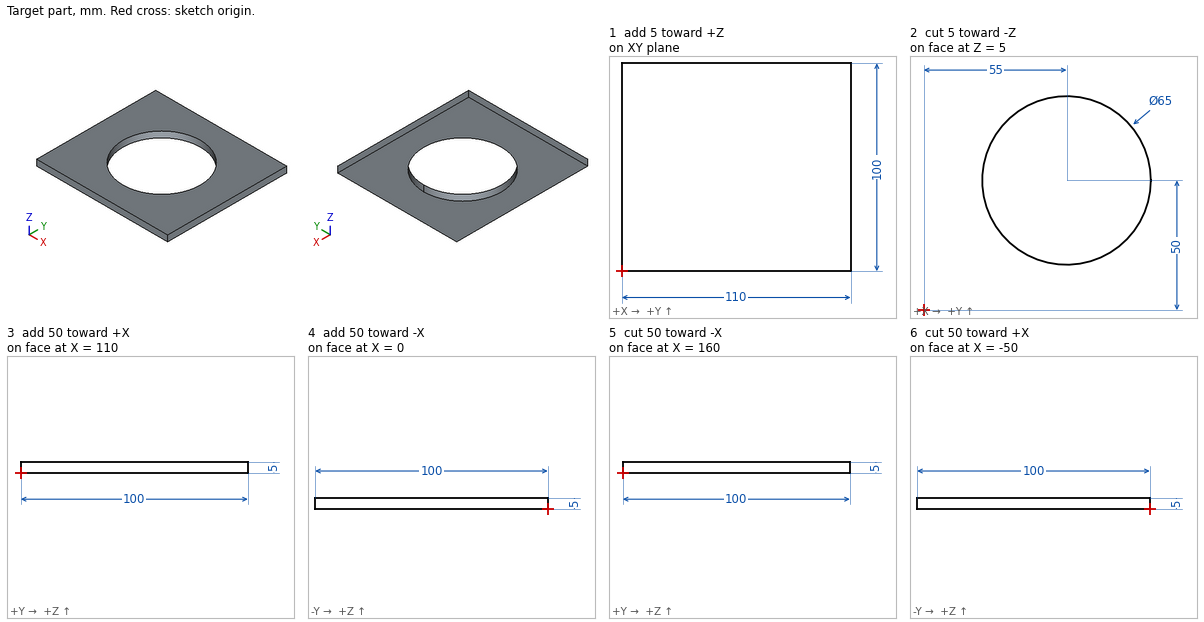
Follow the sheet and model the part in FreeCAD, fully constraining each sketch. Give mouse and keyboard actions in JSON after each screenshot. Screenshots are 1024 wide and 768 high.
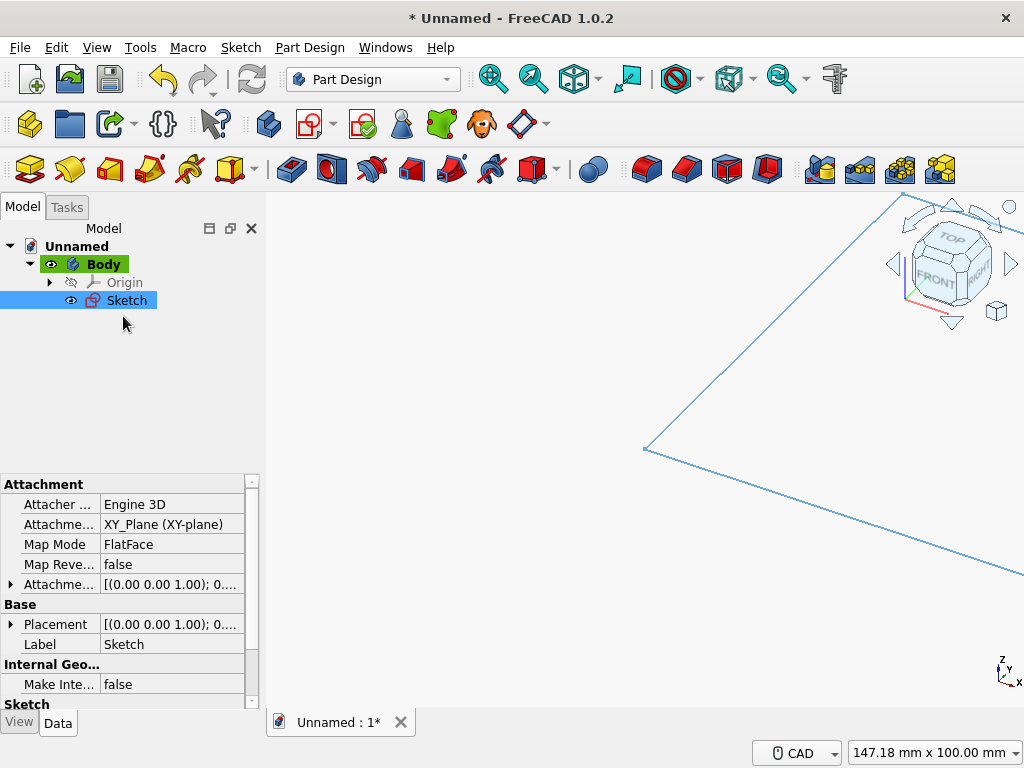
{"action": "left_click", "coordinate": [30, 170]}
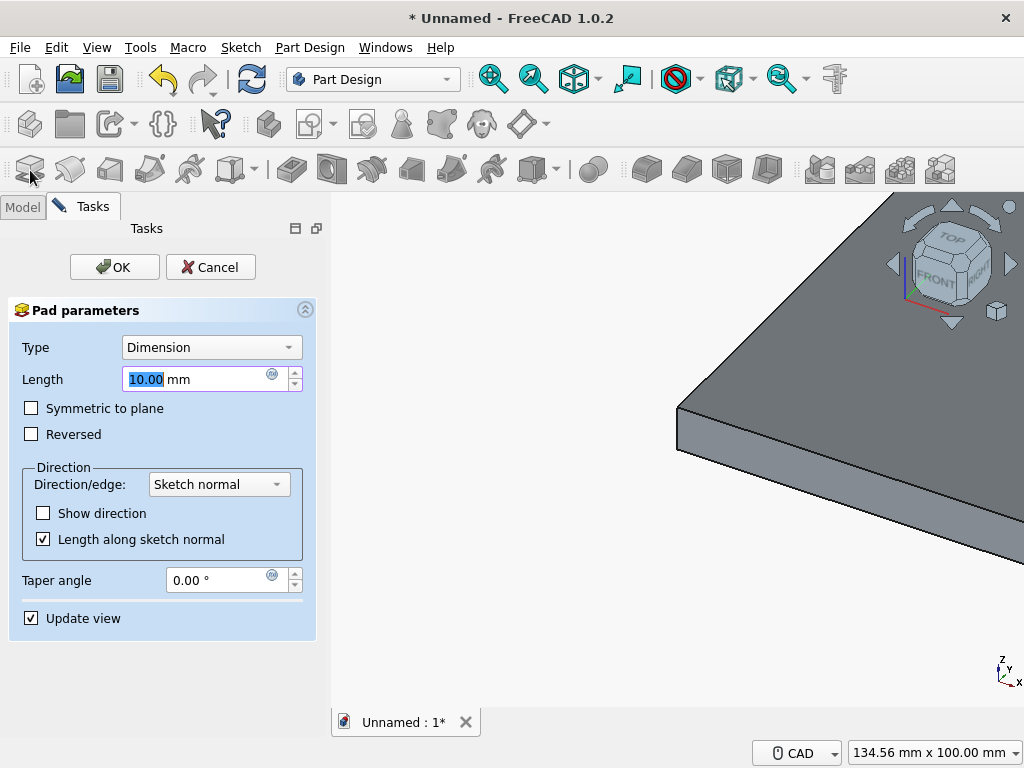
{"action": "type", "text": "5"}
{"action": "key", "text": "Tab"}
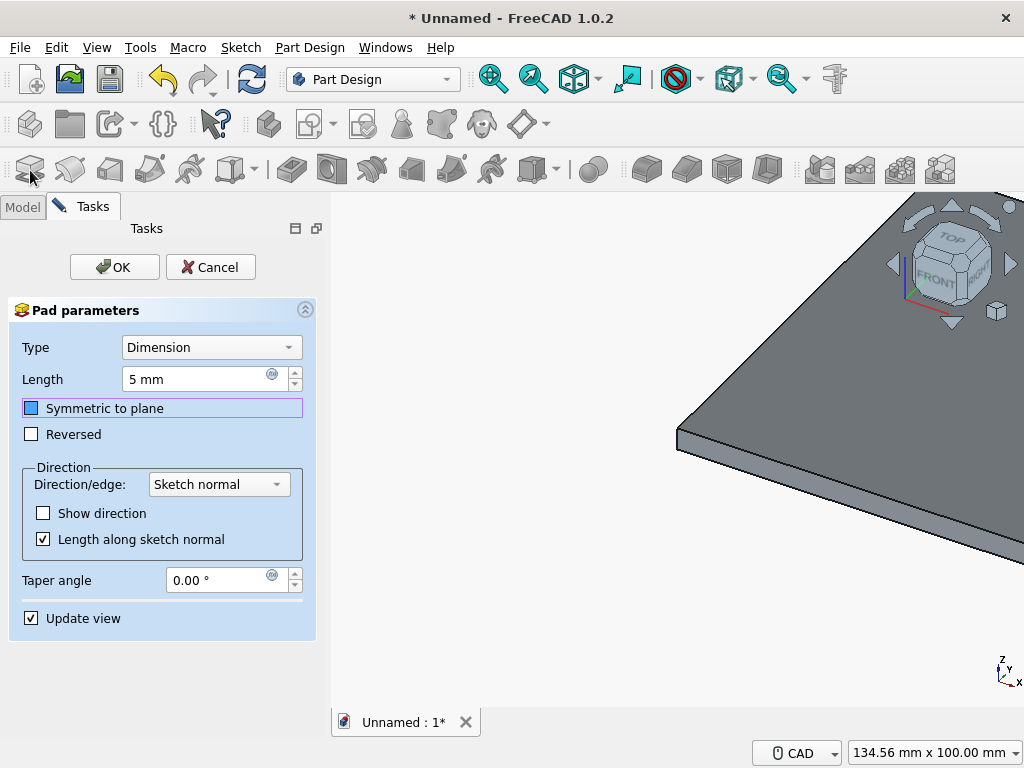
{"action": "left_click", "coordinate": [115, 267]}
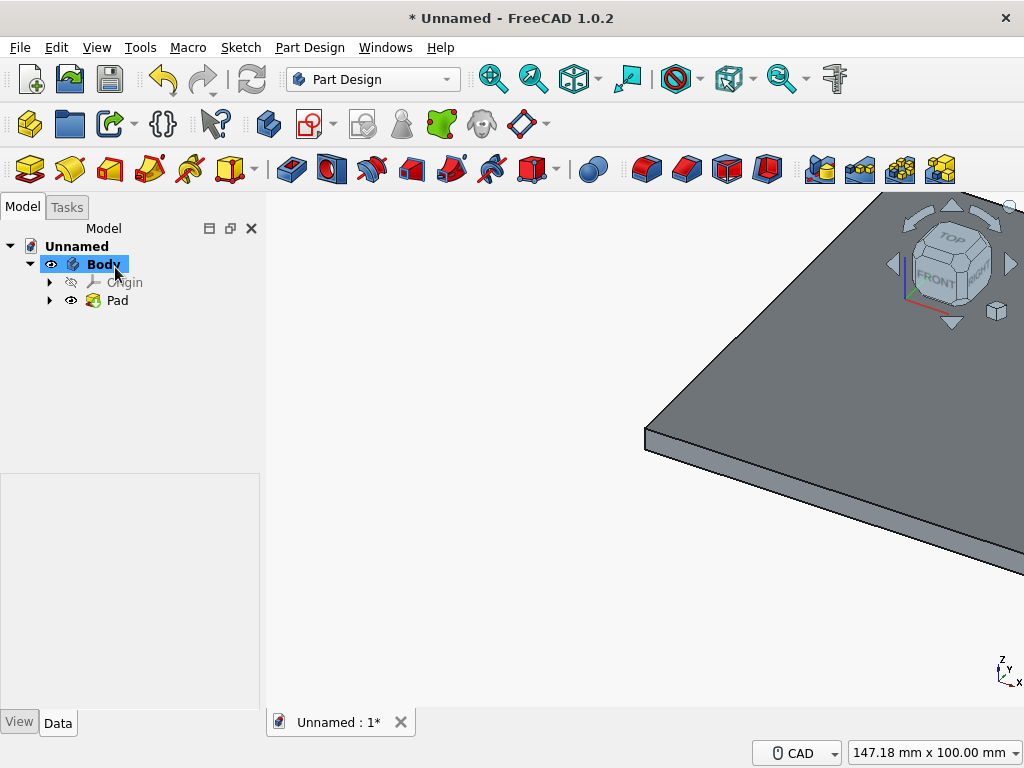
{"action": "left_click", "coordinate": [494, 80]}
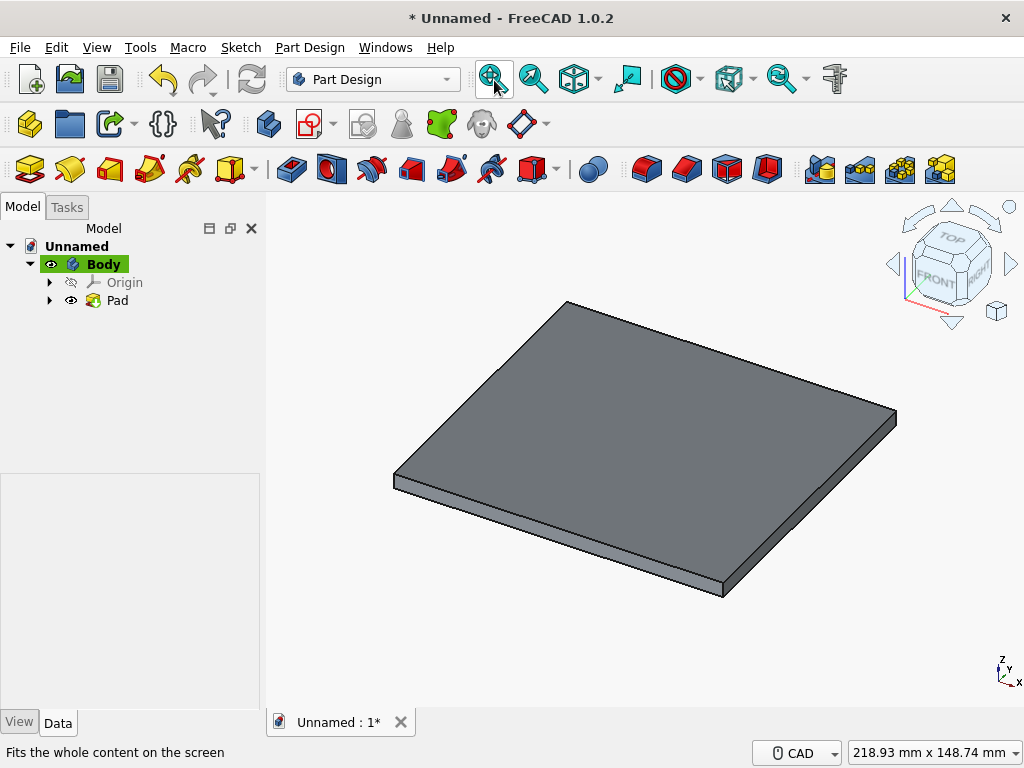
{"action": "left_click", "coordinate": [645, 441]}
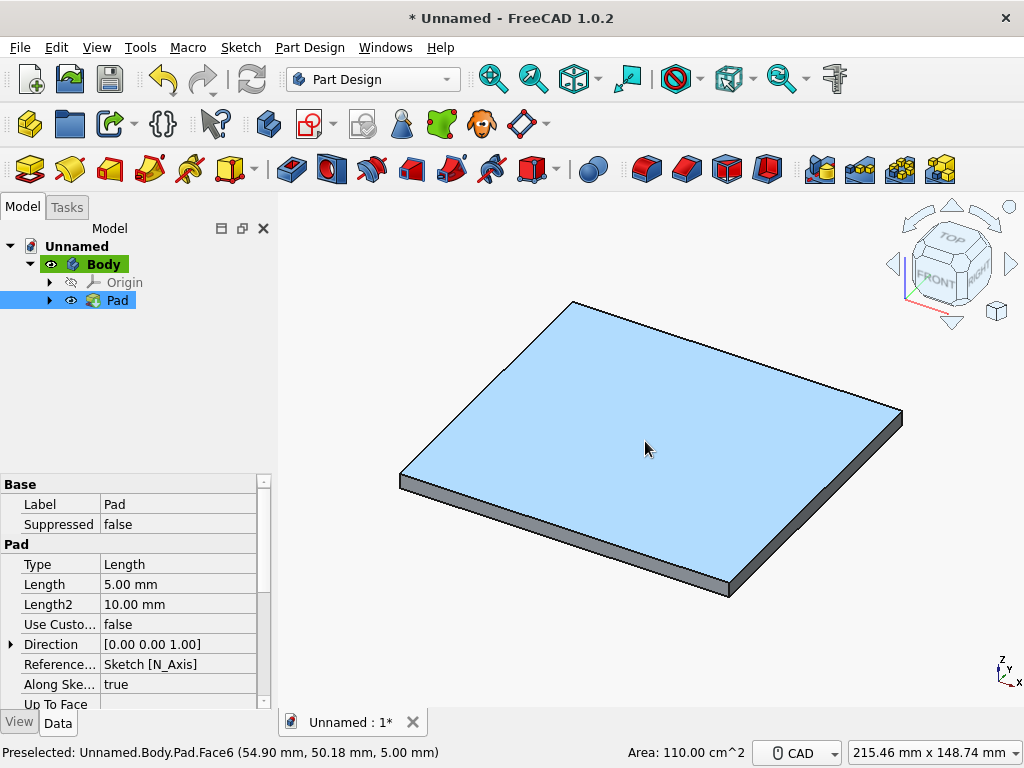
{"action": "left_click", "coordinate": [310, 124]}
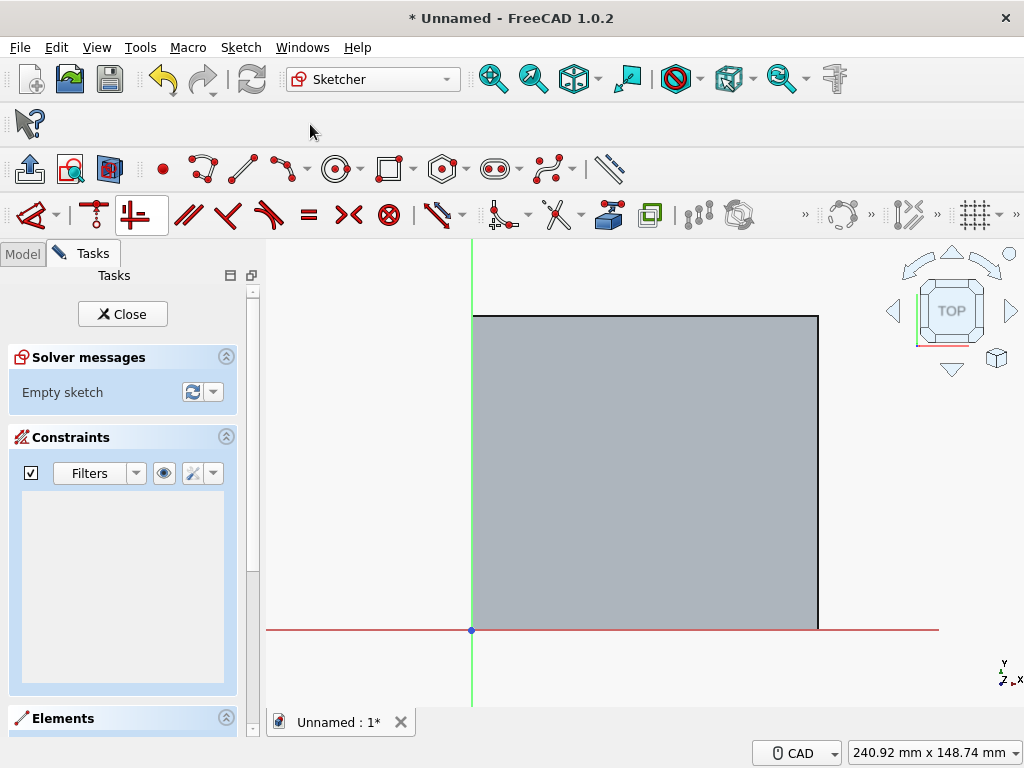
{"action": "left_click", "coordinate": [336, 170]}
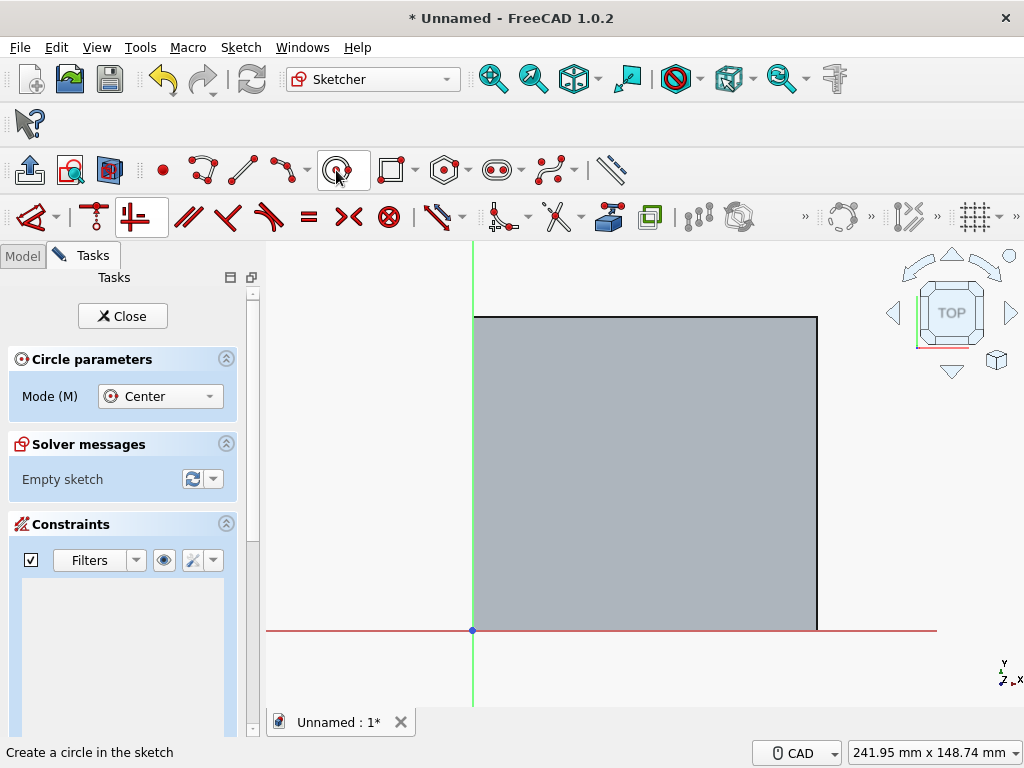
{"action": "left_click", "coordinate": [645, 474]}
{"action": "left_click", "coordinate": [717, 402]}
{"action": "key", "text": "Escape"}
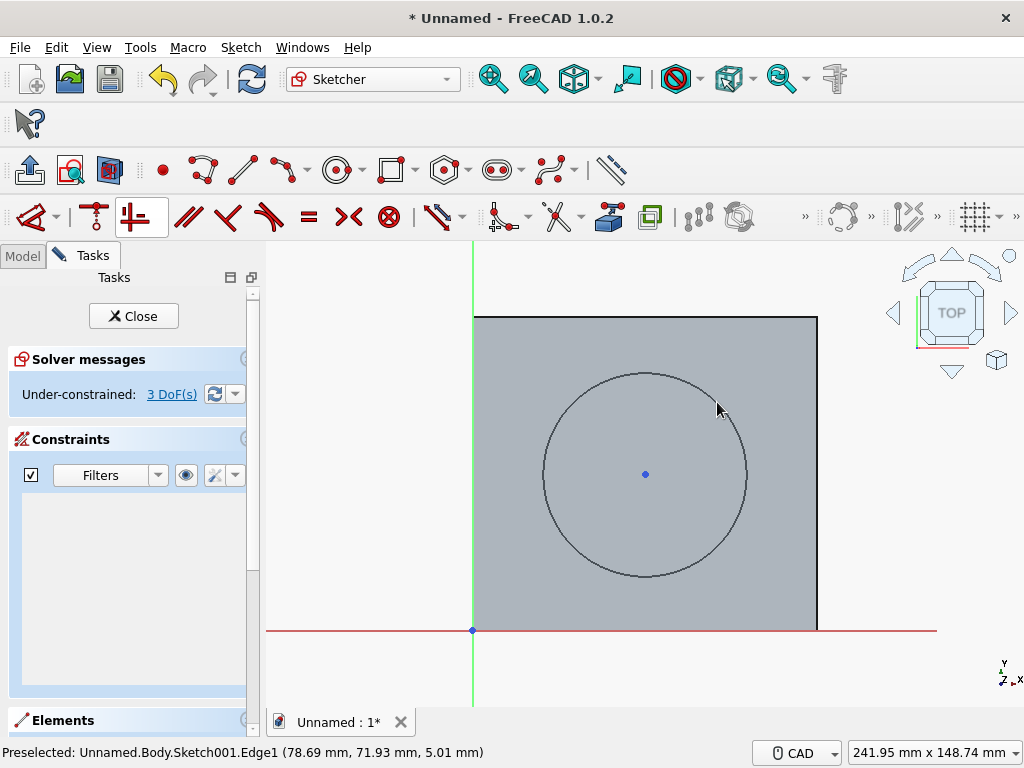
{"action": "left_click", "coordinate": [32, 218]}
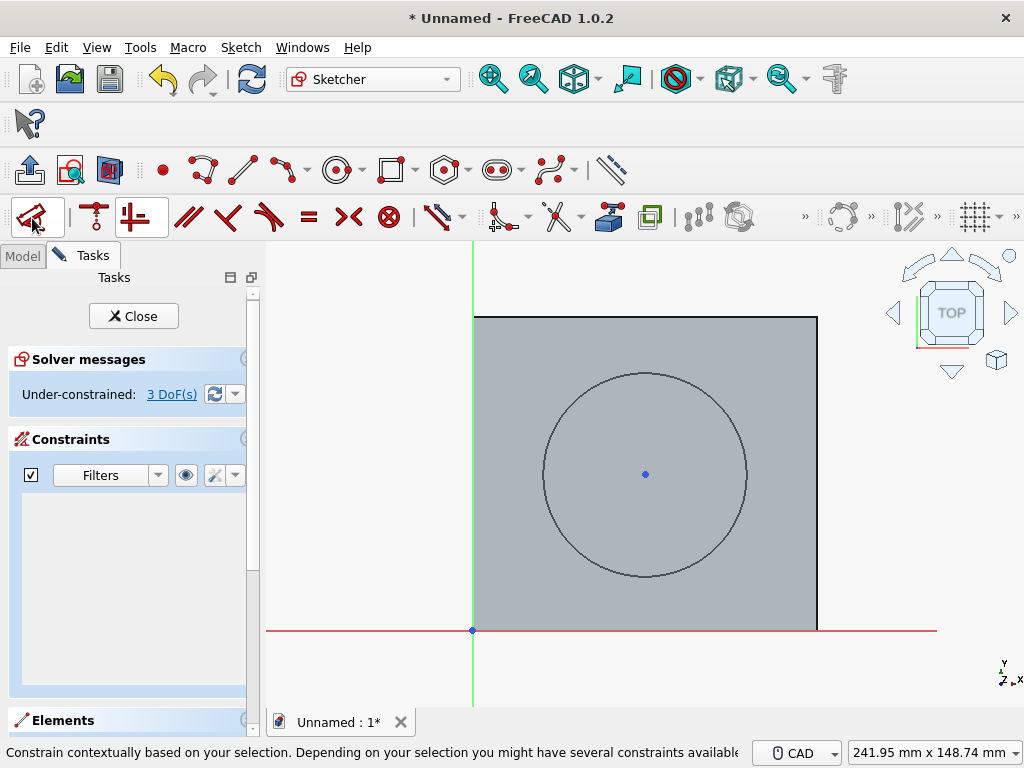
{"action": "left_click", "coordinate": [717, 403]}
{"action": "left_click", "coordinate": [740, 380]}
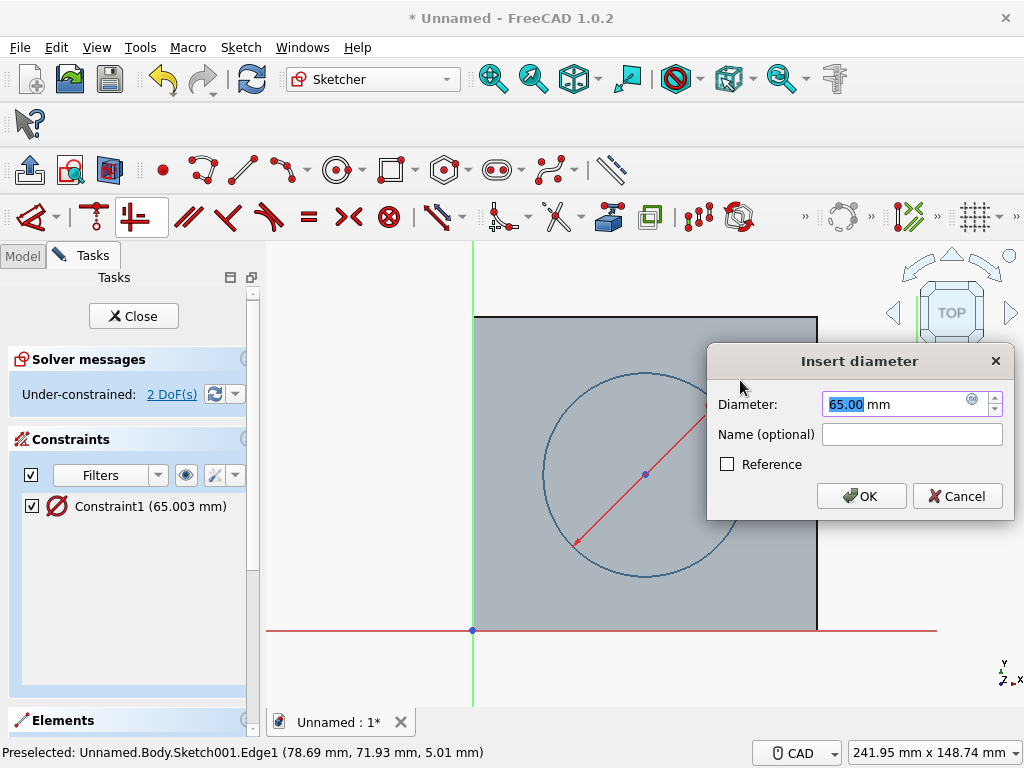
{"action": "type", "text": "65"}
{"action": "key", "text": "Return"}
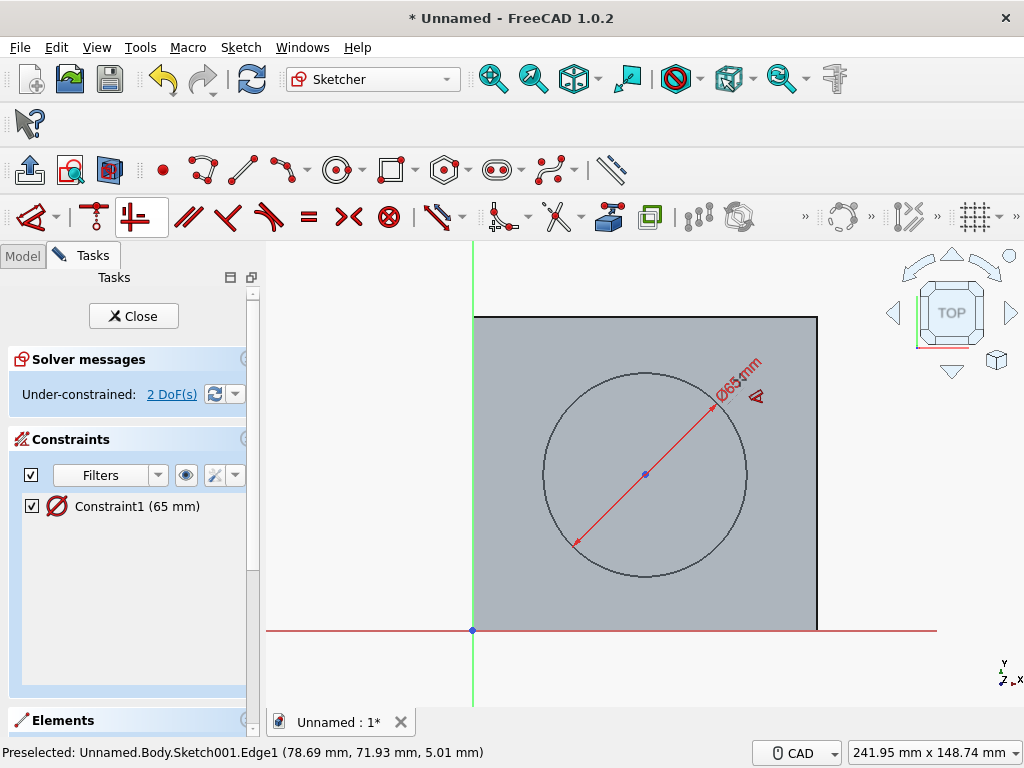
{"action": "left_click", "coordinate": [645, 475]}
{"action": "left_click", "coordinate": [559, 665]}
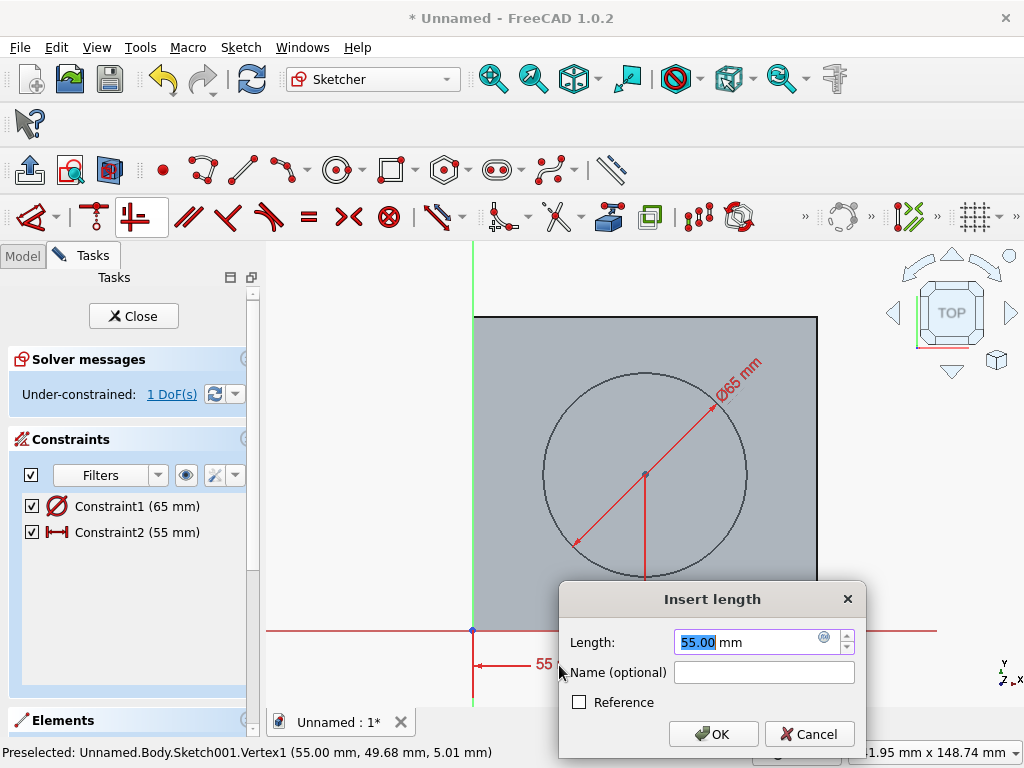
{"action": "type", "text": "55"}
{"action": "key", "text": "Return"}